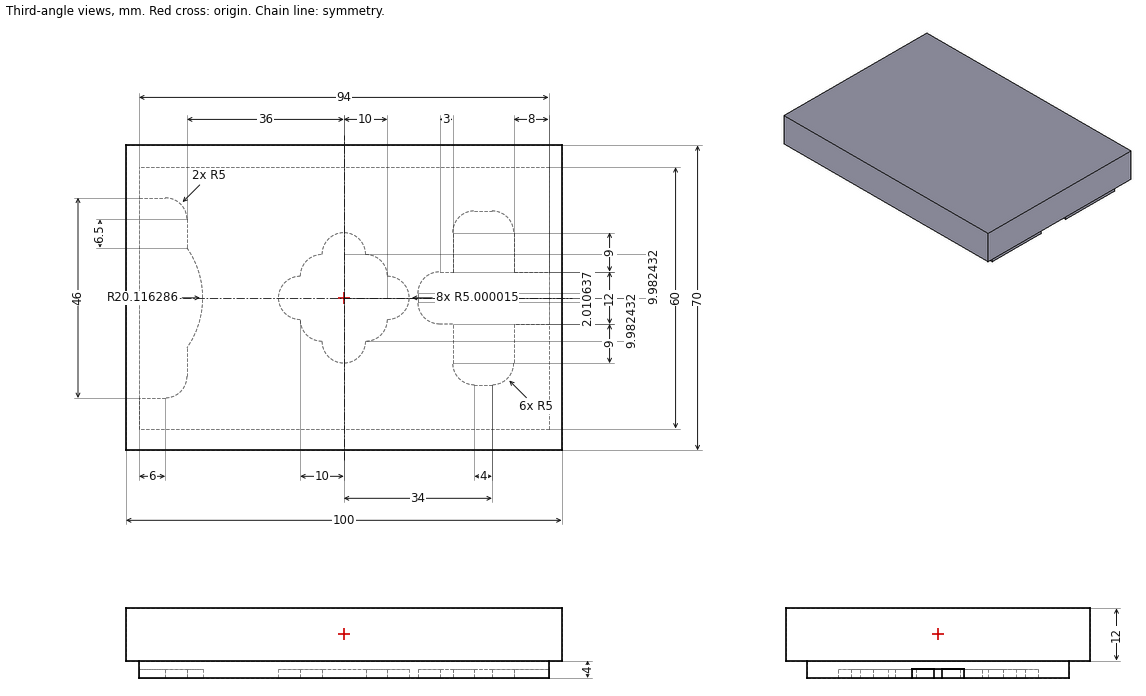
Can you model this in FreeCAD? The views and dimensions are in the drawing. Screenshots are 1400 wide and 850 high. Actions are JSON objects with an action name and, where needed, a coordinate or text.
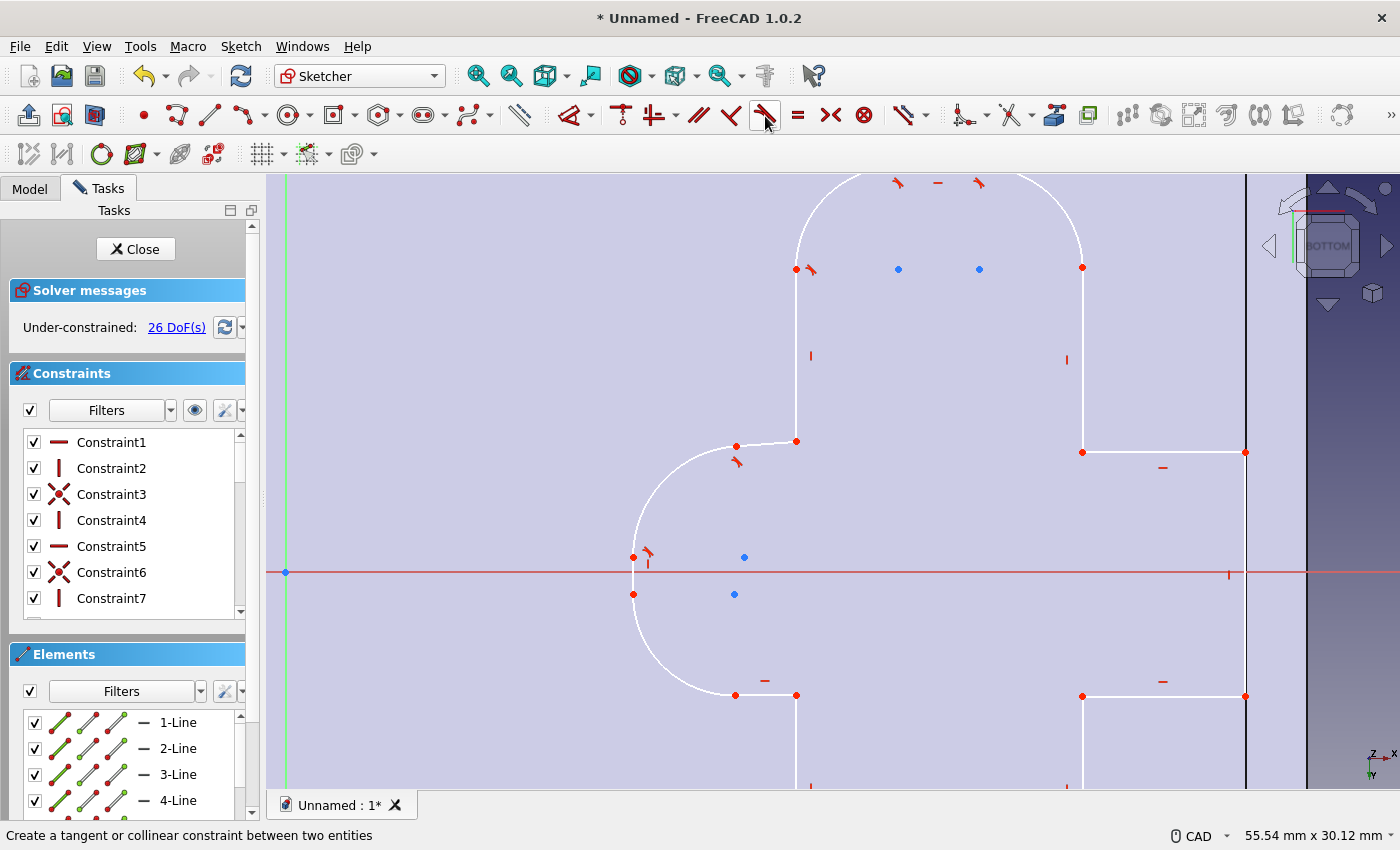
{"action": "scroll", "coordinate": [633, 568], "scroll_direction": "up", "scroll_amount": 2}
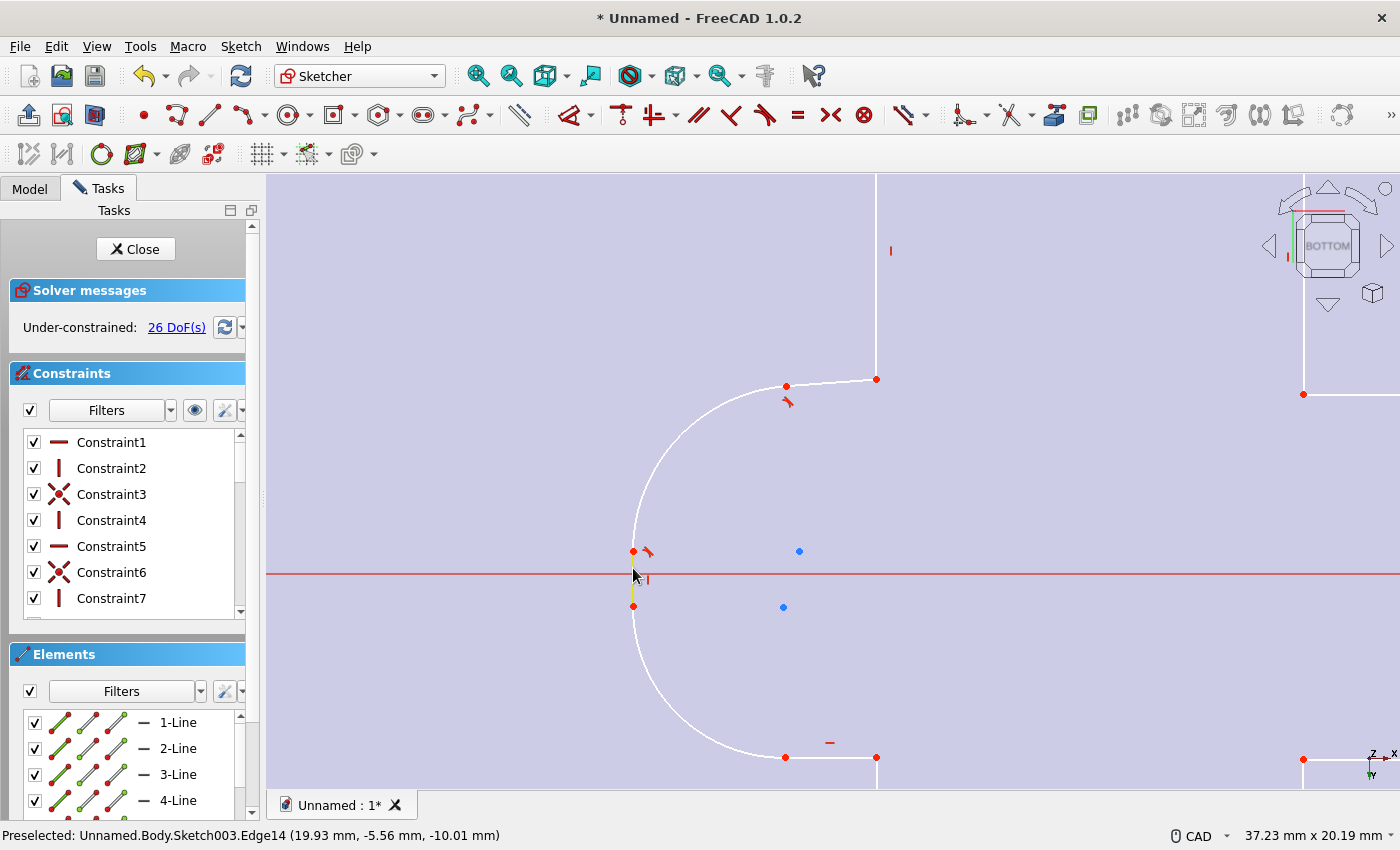
{"action": "left_click", "coordinate": [633, 568]}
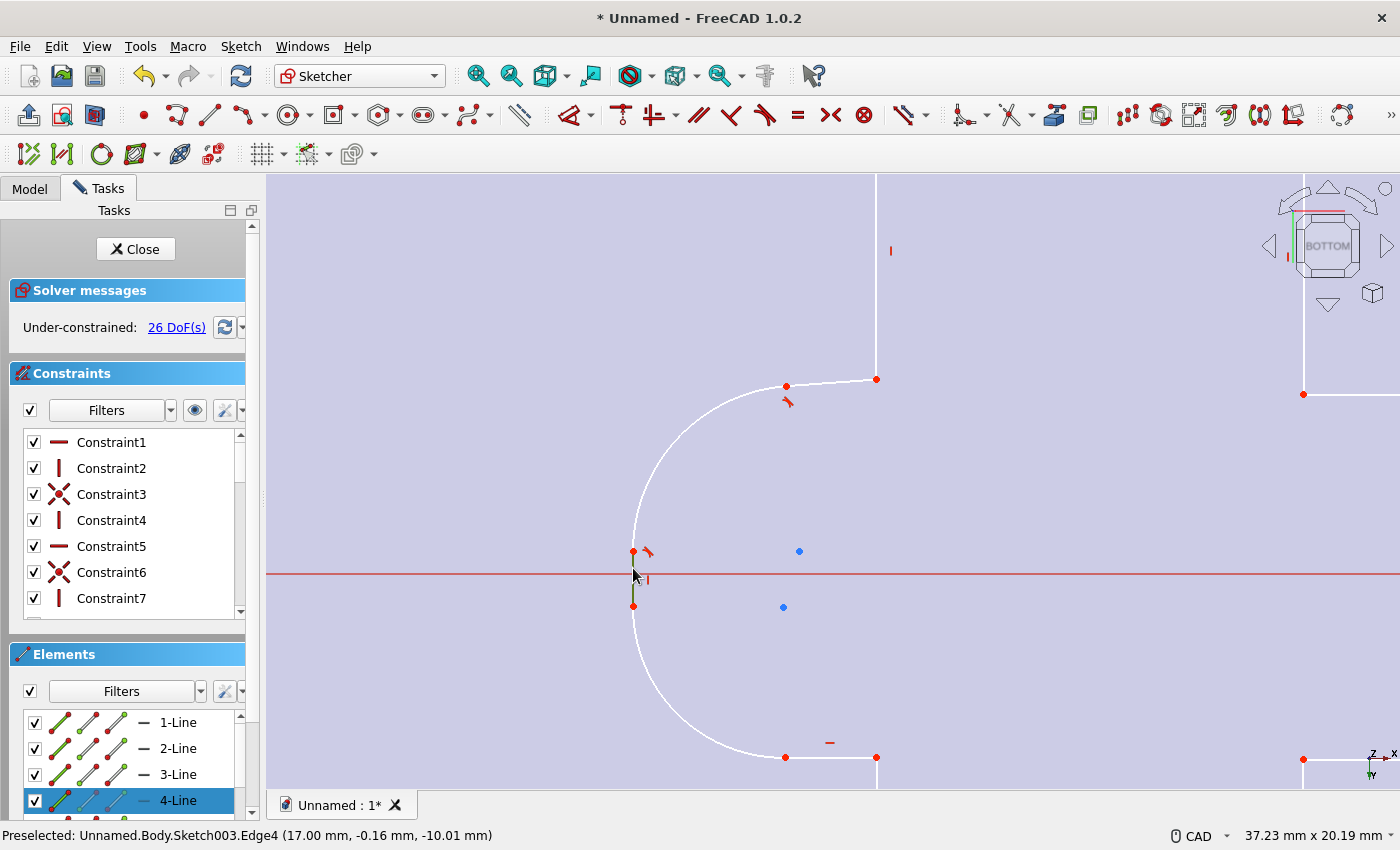
{"action": "left_click", "coordinate": [649, 676]}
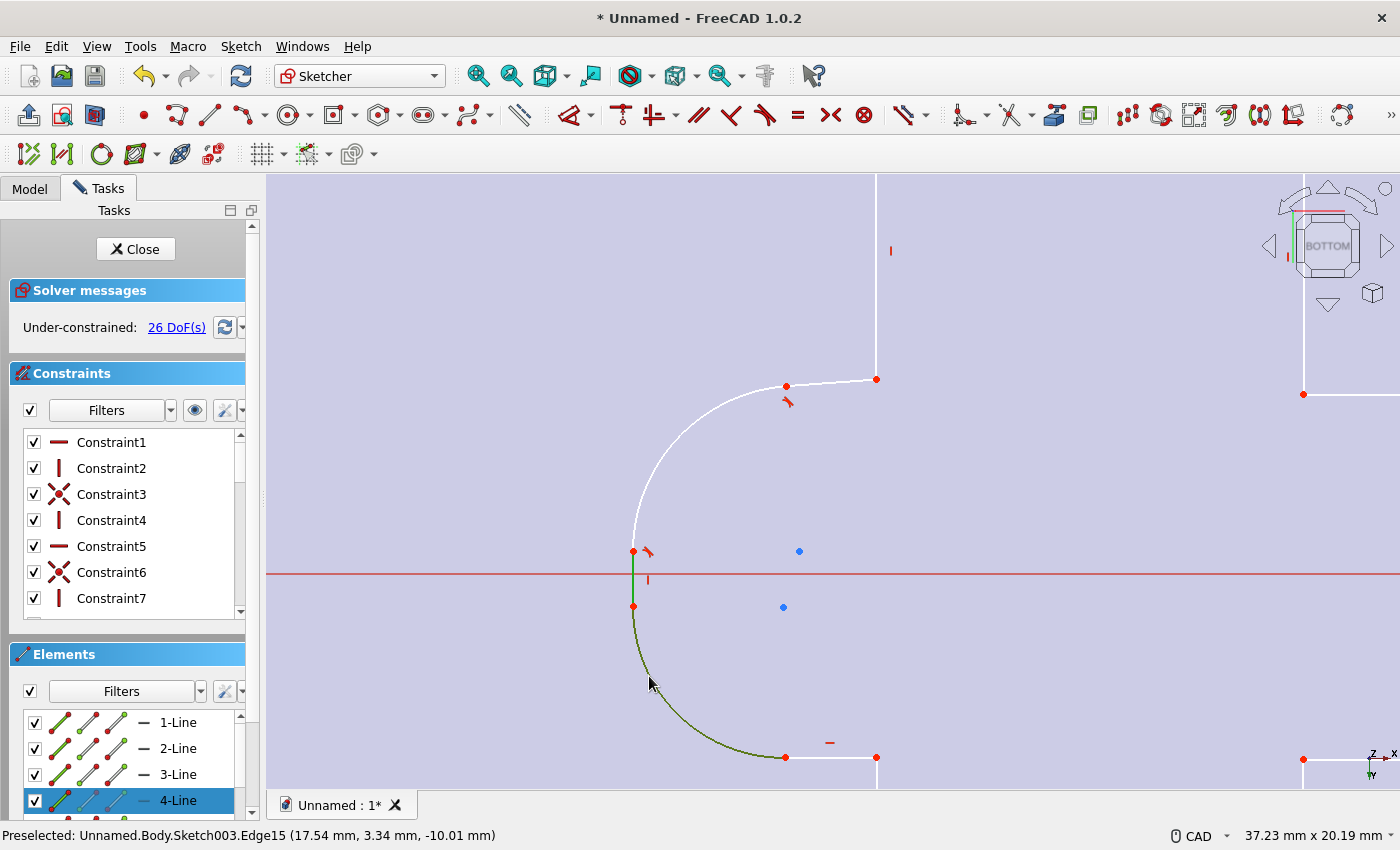
{"action": "left_click", "coordinate": [765, 116]}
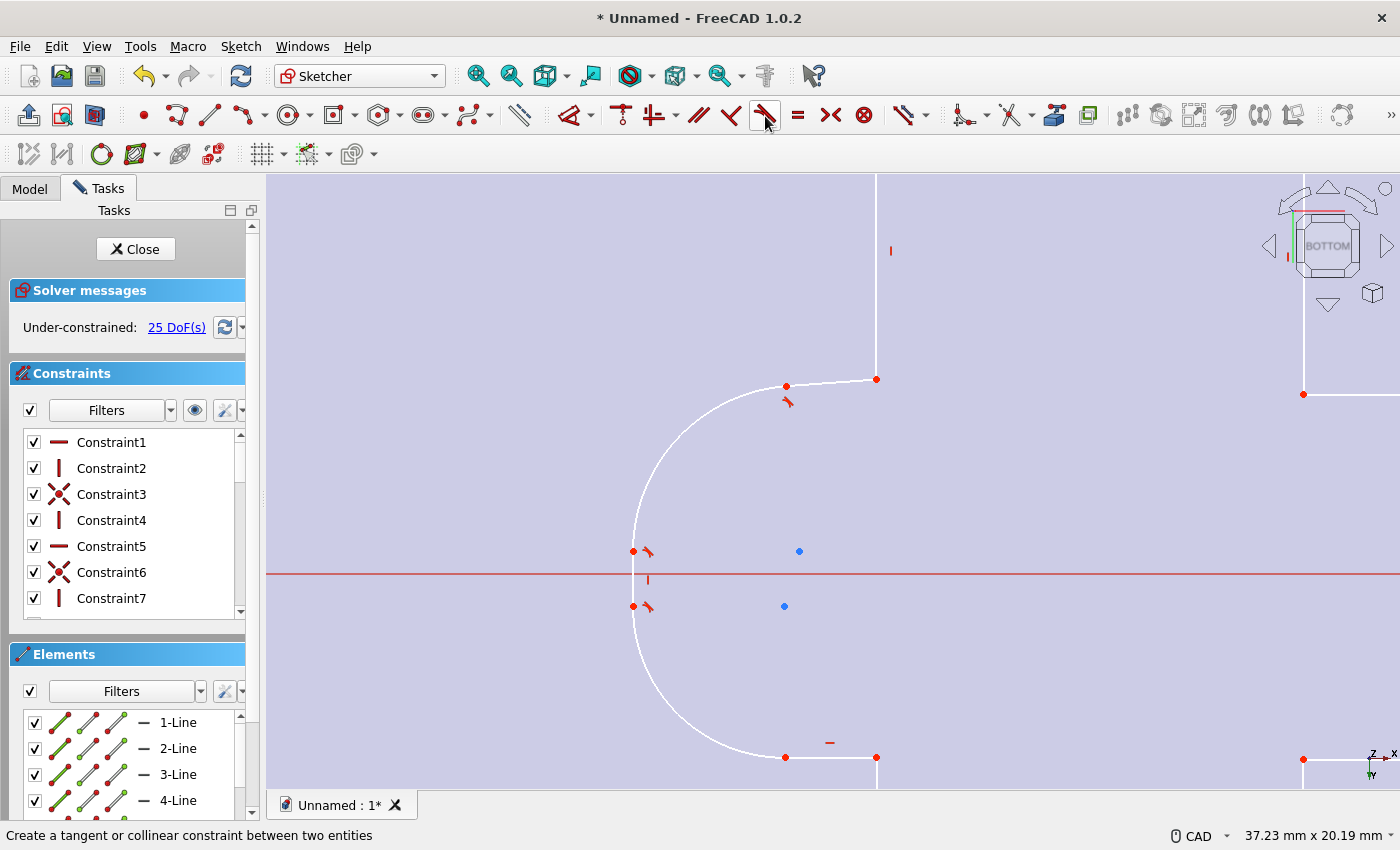
{"action": "left_click", "coordinate": [813, 758]}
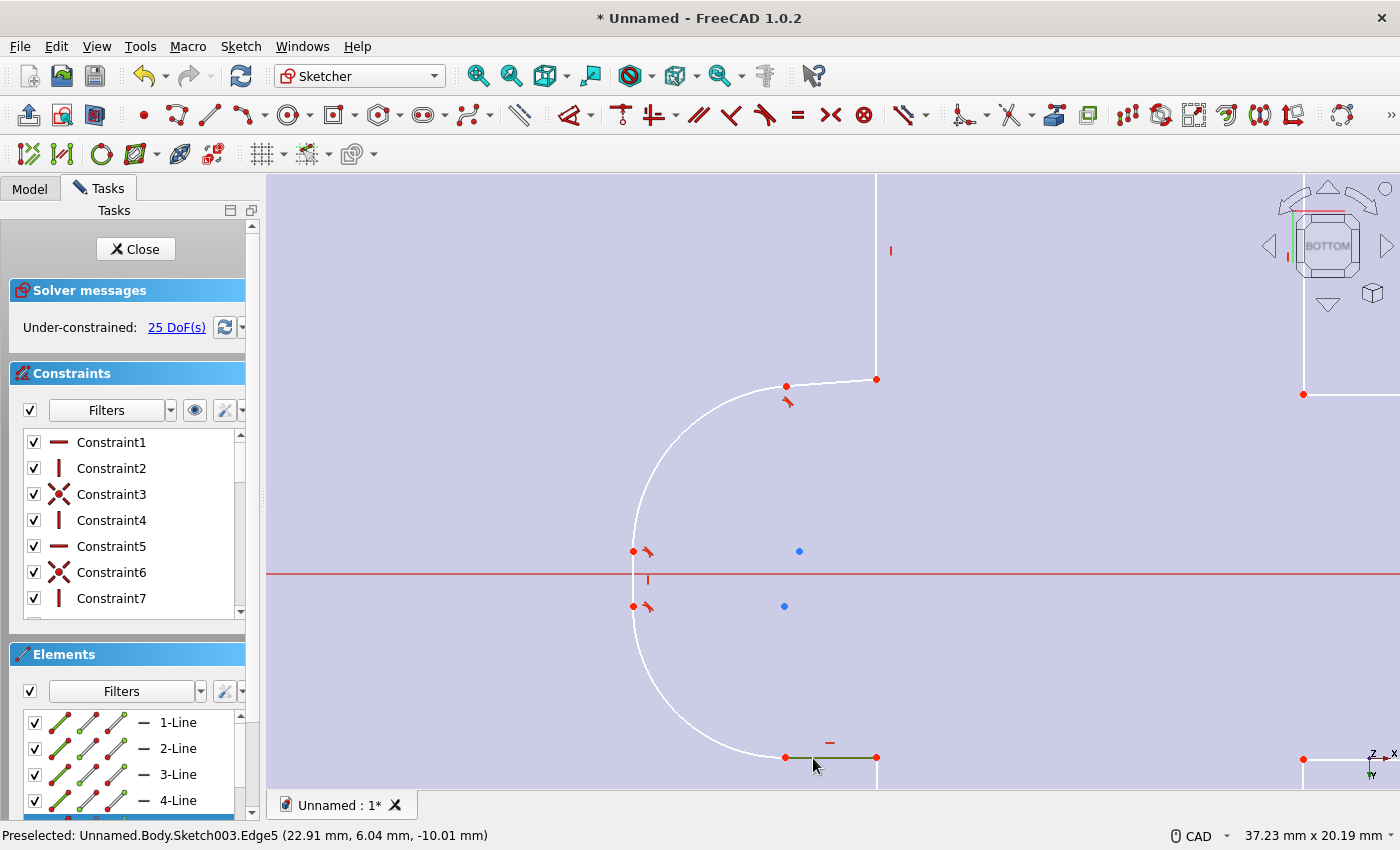
{"action": "left_click", "coordinate": [650, 676]}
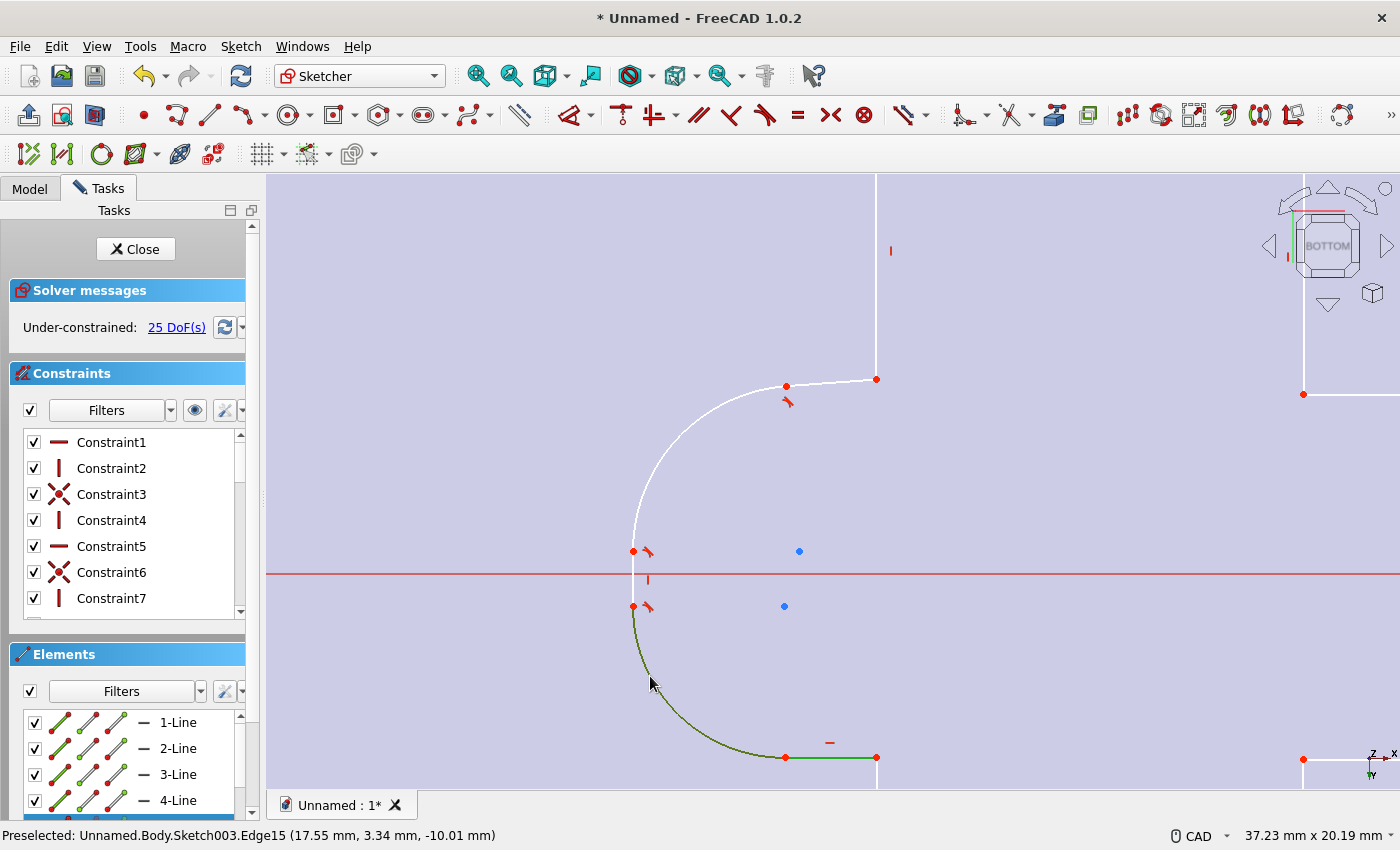
{"action": "left_click", "coordinate": [765, 116]}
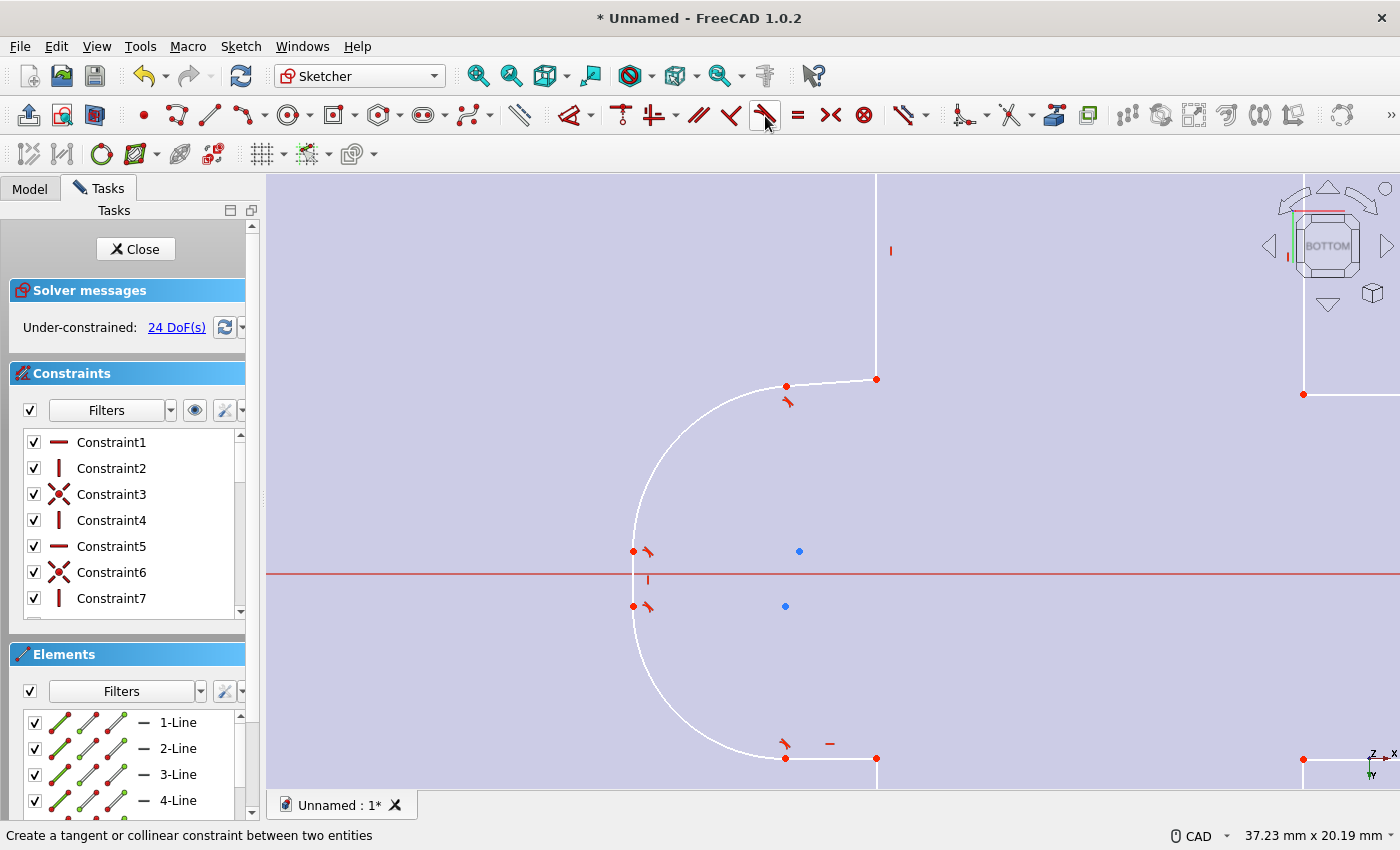
{"action": "scroll", "coordinate": [736, 442], "scroll_direction": "down", "scroll_amount": 6}